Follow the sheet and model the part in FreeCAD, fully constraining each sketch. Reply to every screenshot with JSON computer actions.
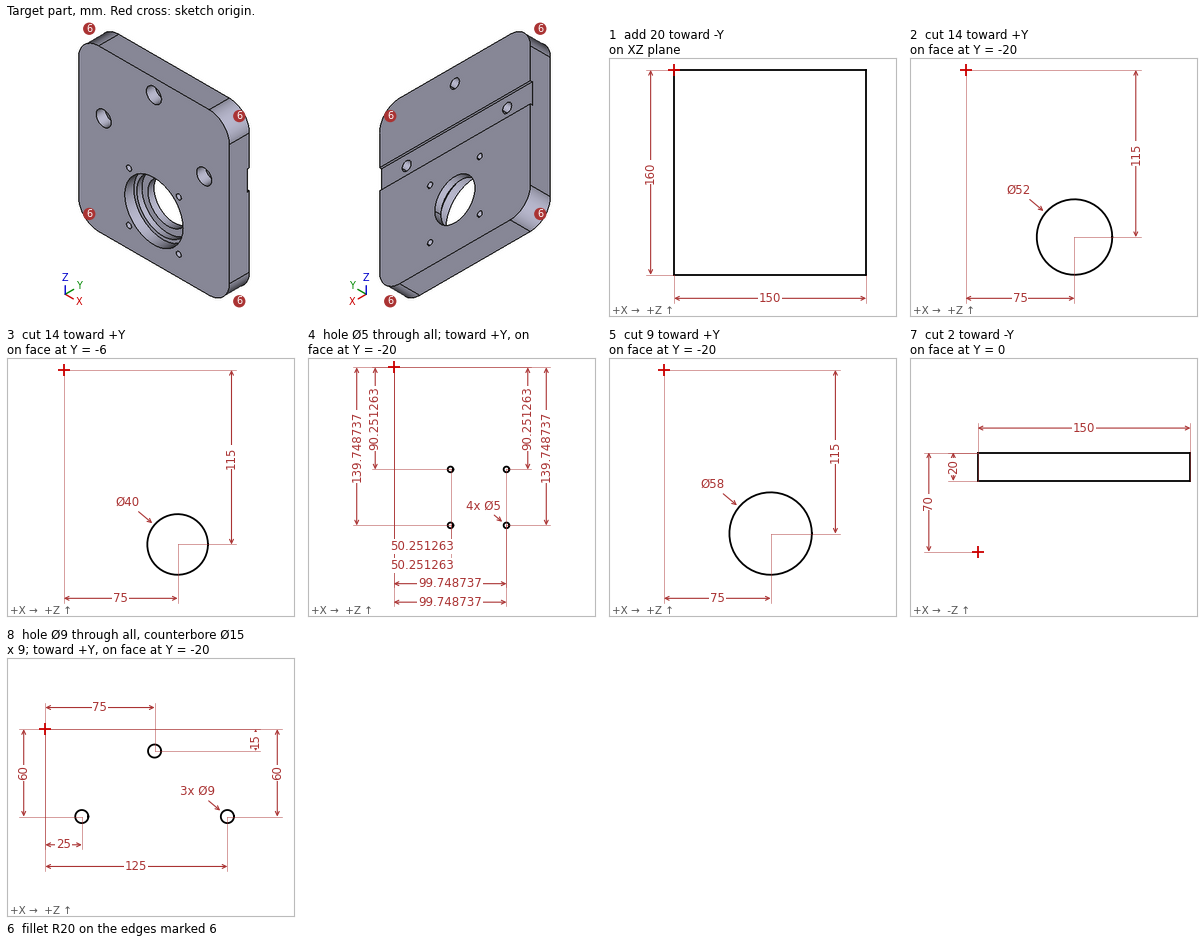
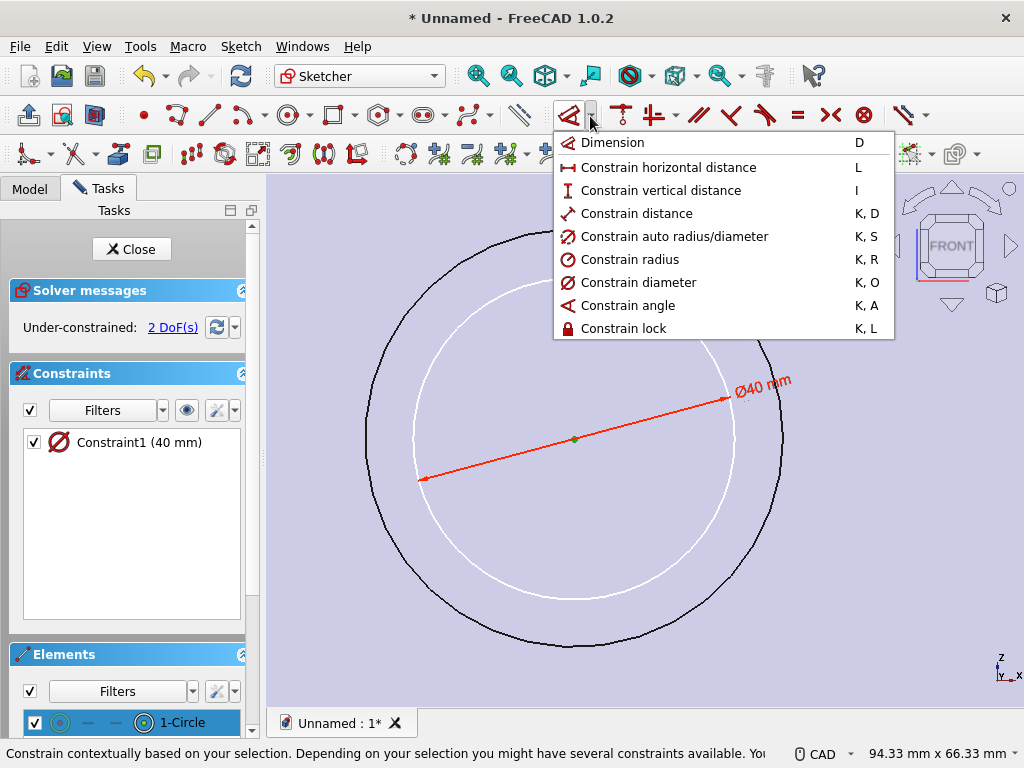
{"action": "left_click", "coordinate": [724, 168]}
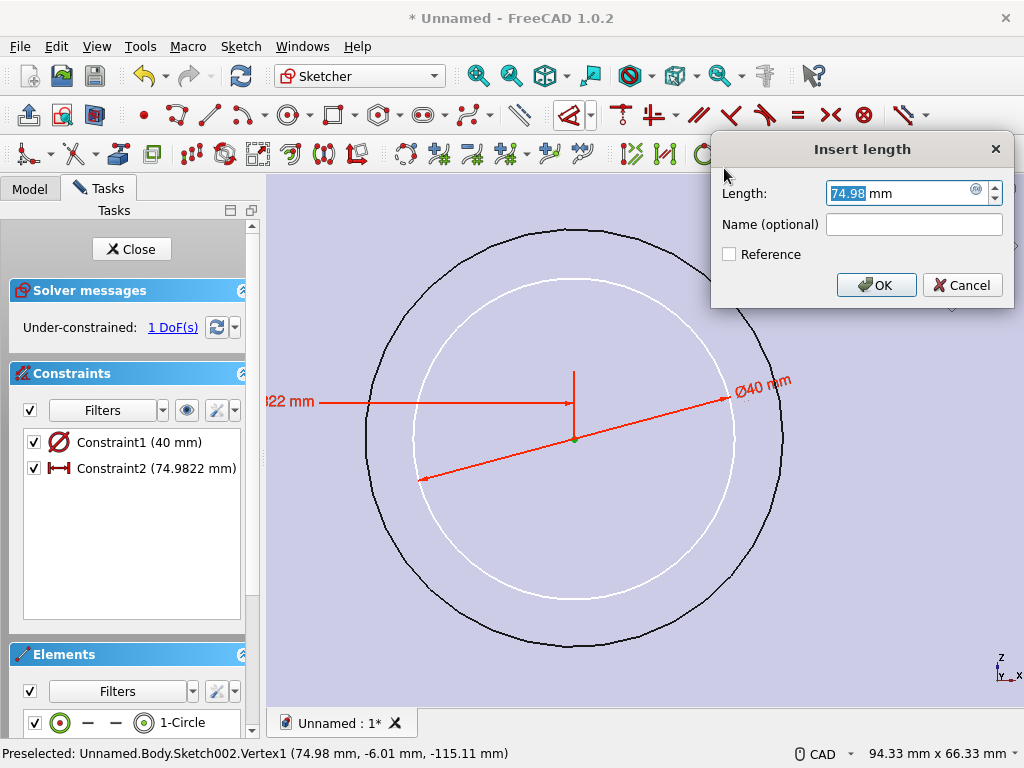
{"action": "type", "text": "75"}
{"action": "key", "text": "Return"}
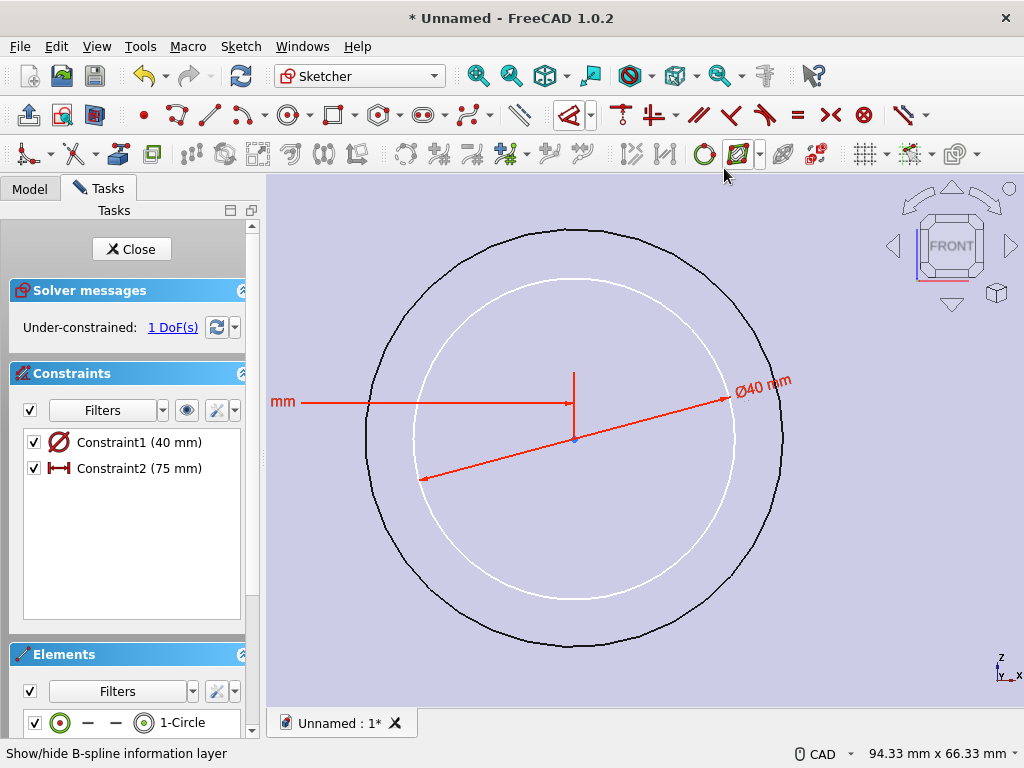
{"action": "left_click", "coordinate": [574, 439]}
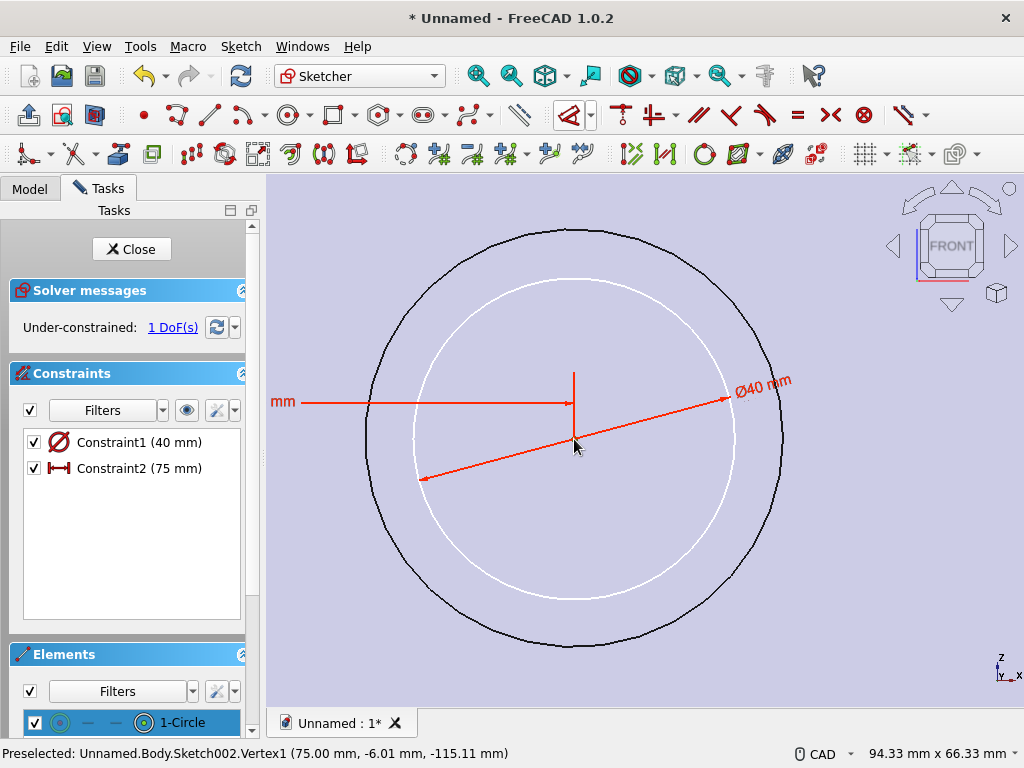
{"action": "key", "text": "i"}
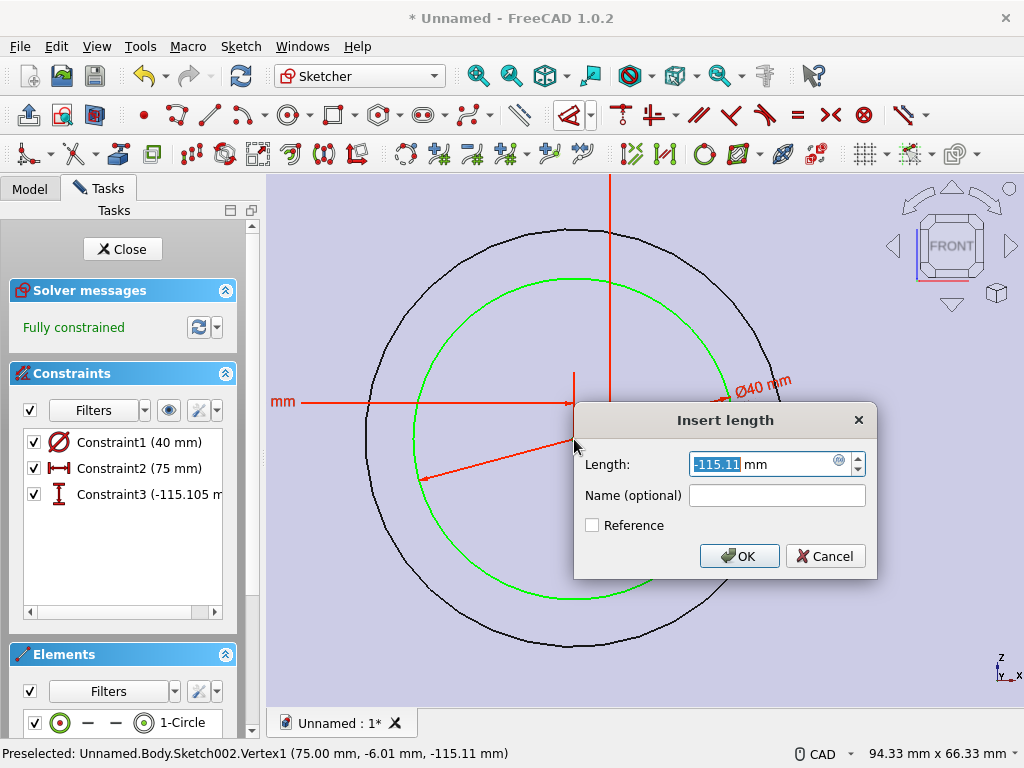
{"action": "type", "text": "-115"}
{"action": "key", "text": "Return"}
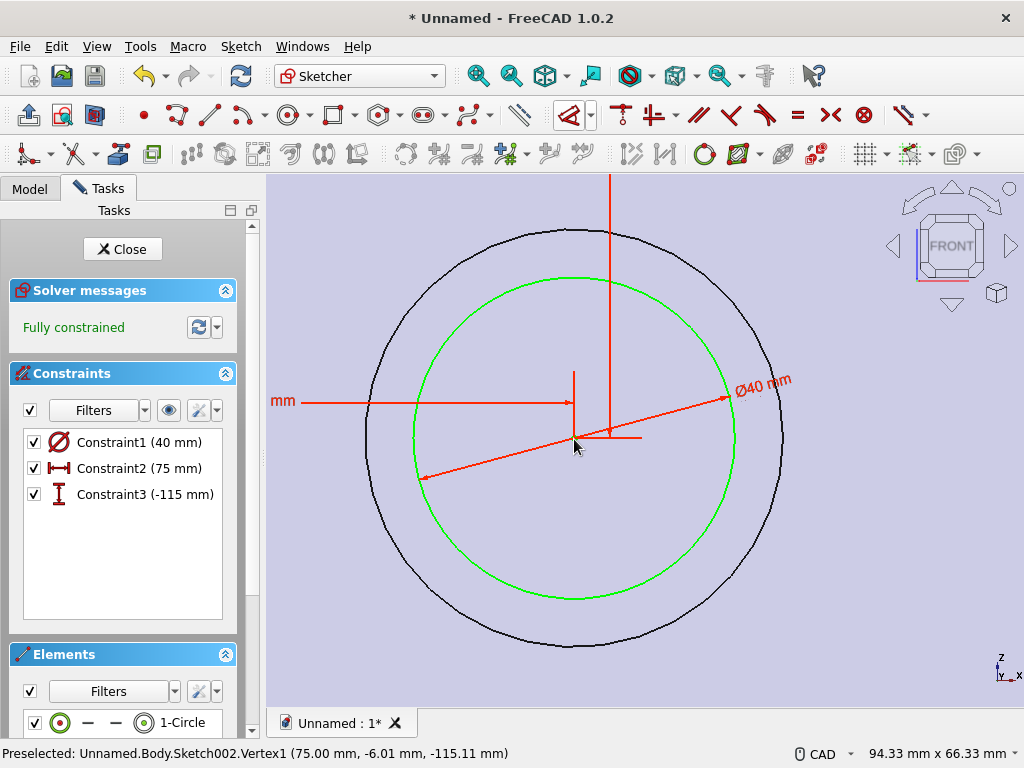
{"action": "left_click", "coordinate": [123, 249]}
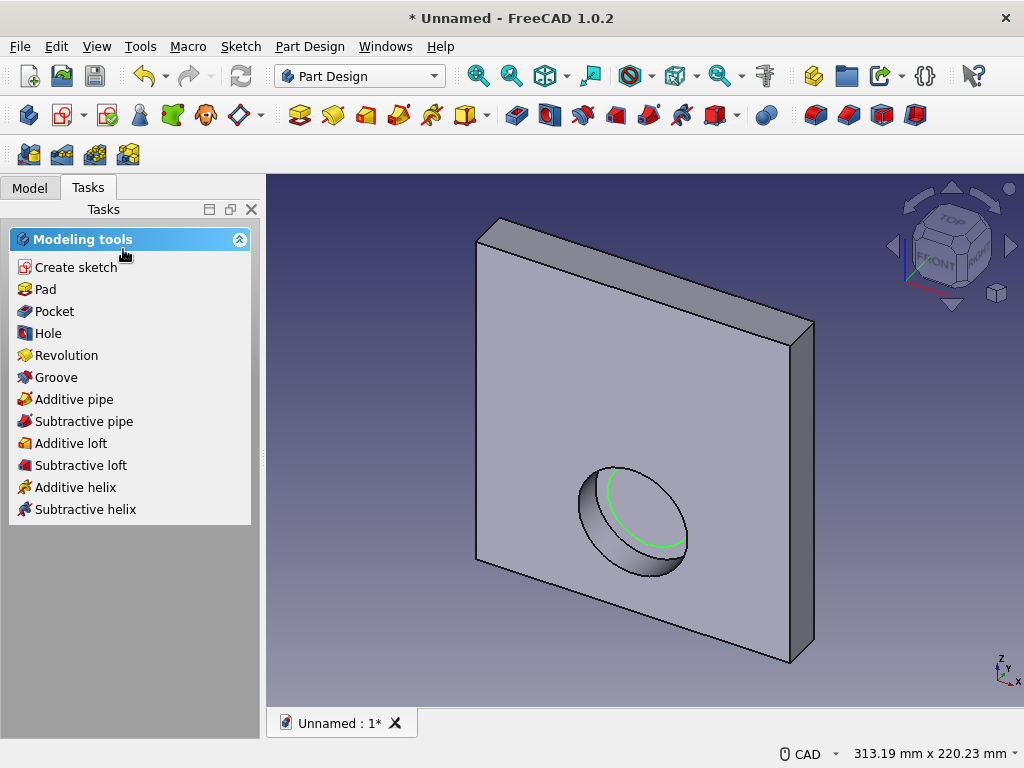
{"action": "left_click", "coordinate": [517, 116]}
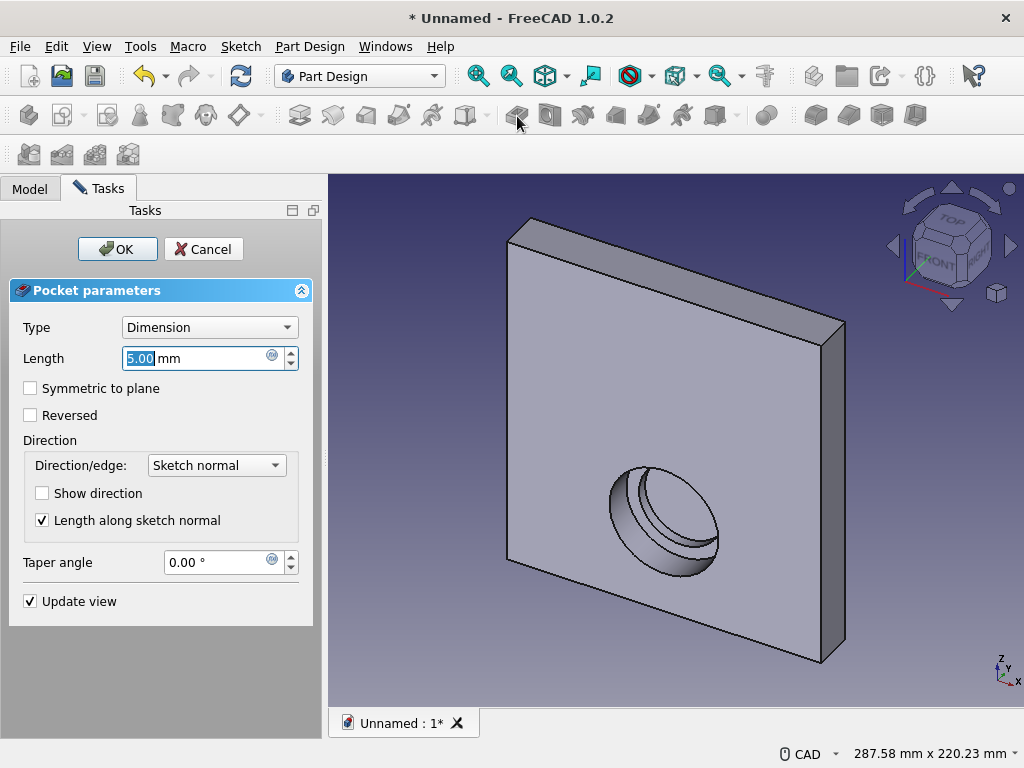
{"action": "type", "text": "14"}
{"action": "key", "text": "Tab"}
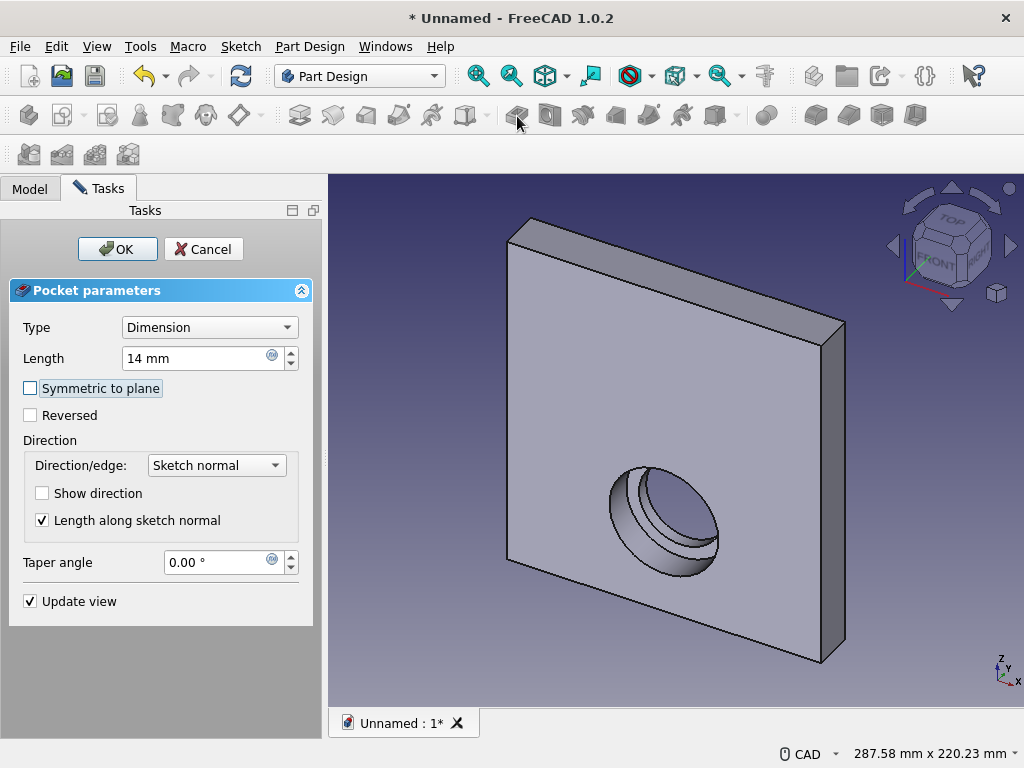
{"action": "left_click", "coordinate": [118, 249]}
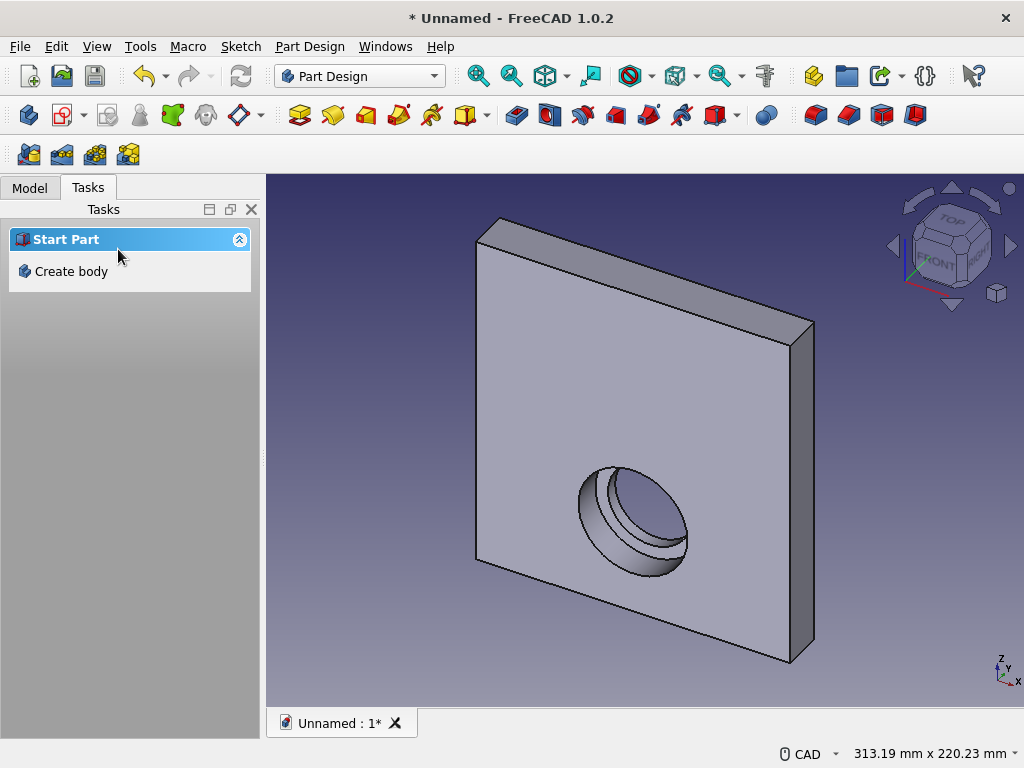
{"action": "left_click", "coordinate": [678, 421]}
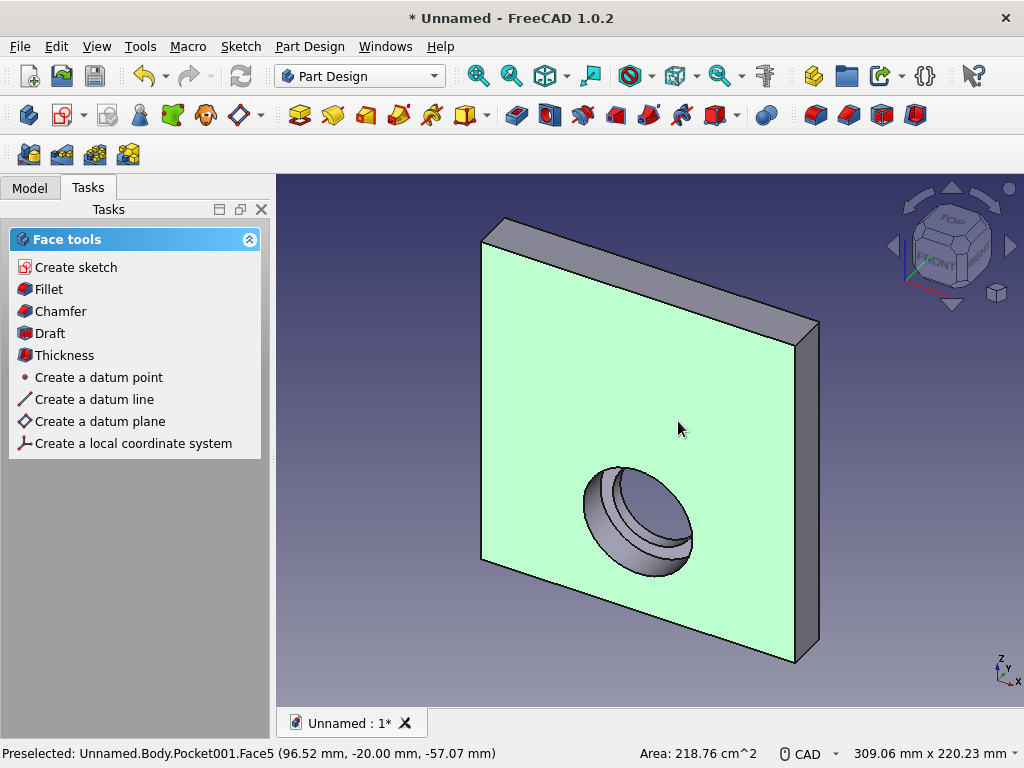
{"action": "left_click", "coordinate": [62, 116]}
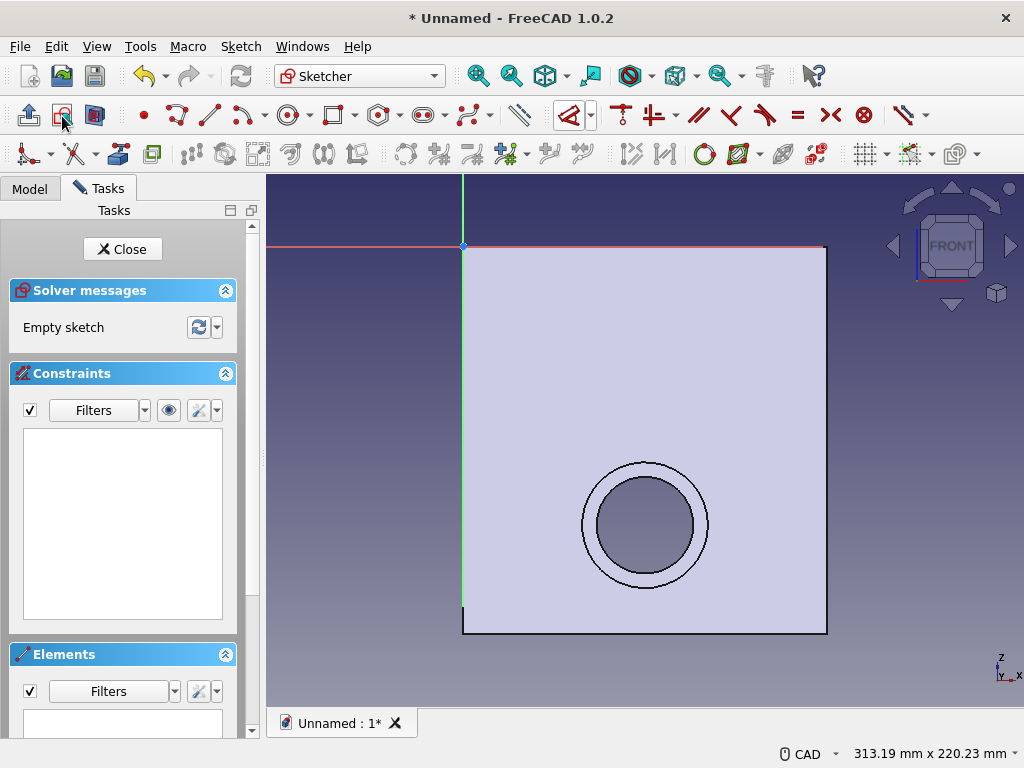
{"action": "scroll", "coordinate": [685, 575], "scroll_direction": "up", "scroll_amount": 5}